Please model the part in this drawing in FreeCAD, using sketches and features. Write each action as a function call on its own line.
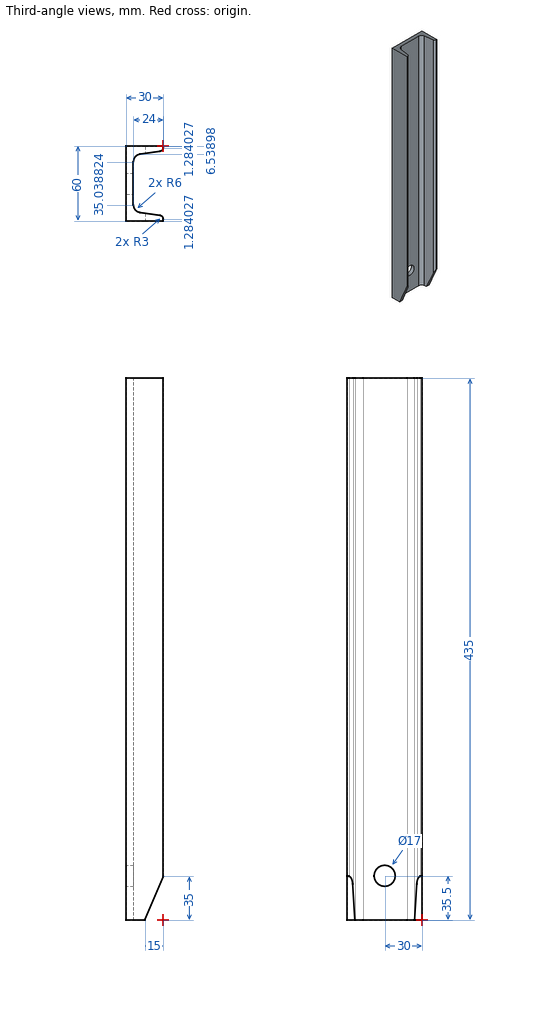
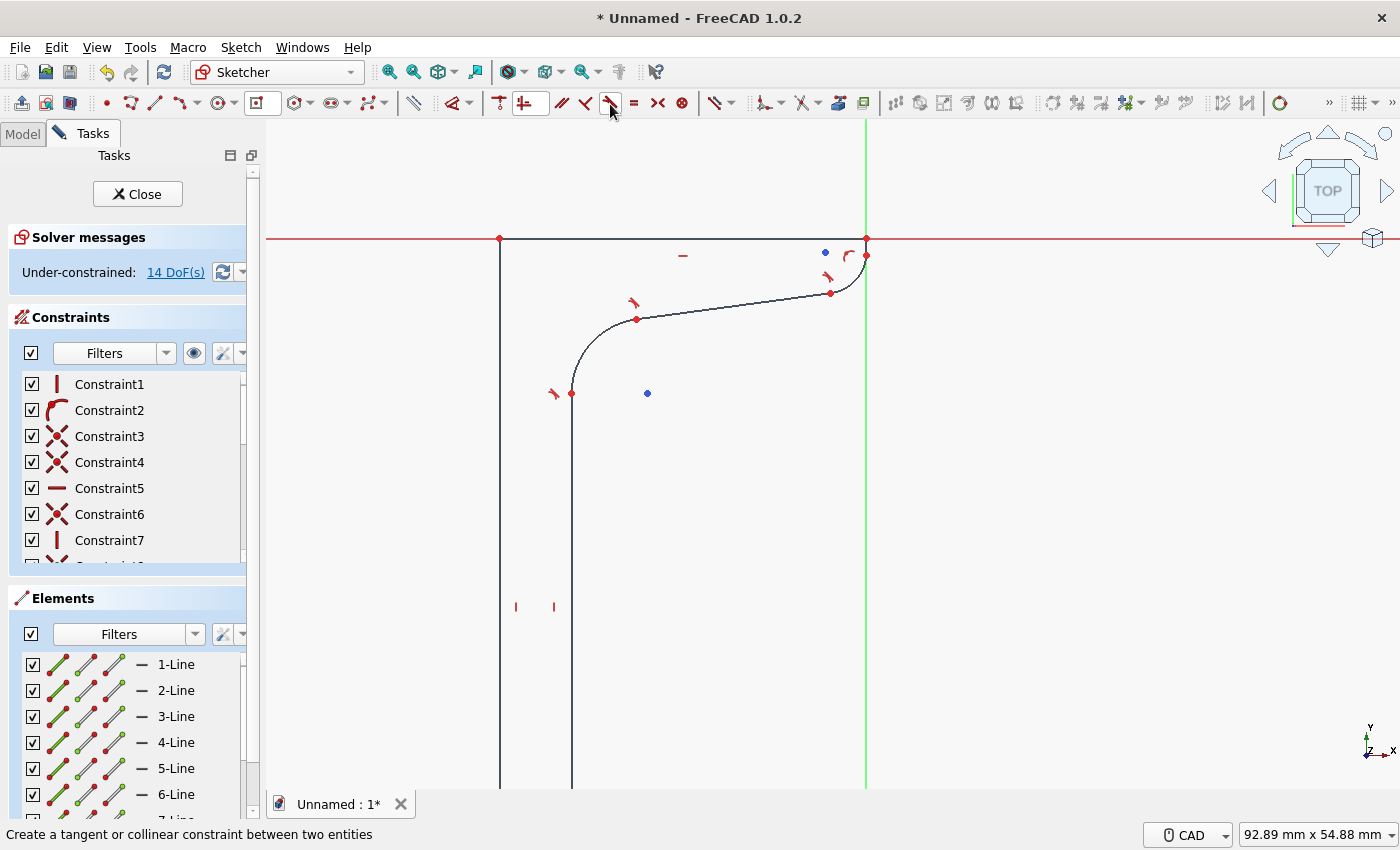
scroll(866, 247, up, 3)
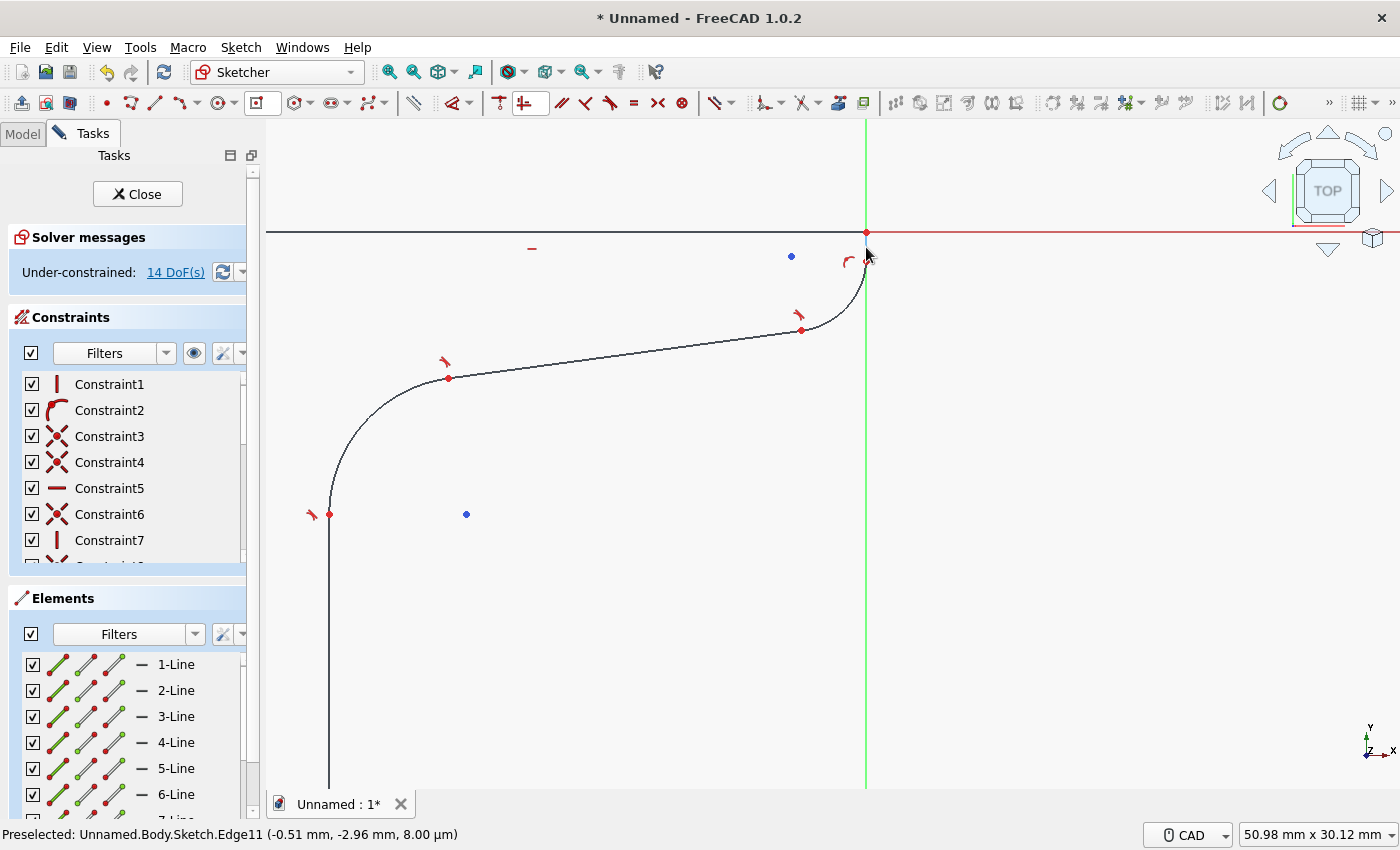
click(866, 247)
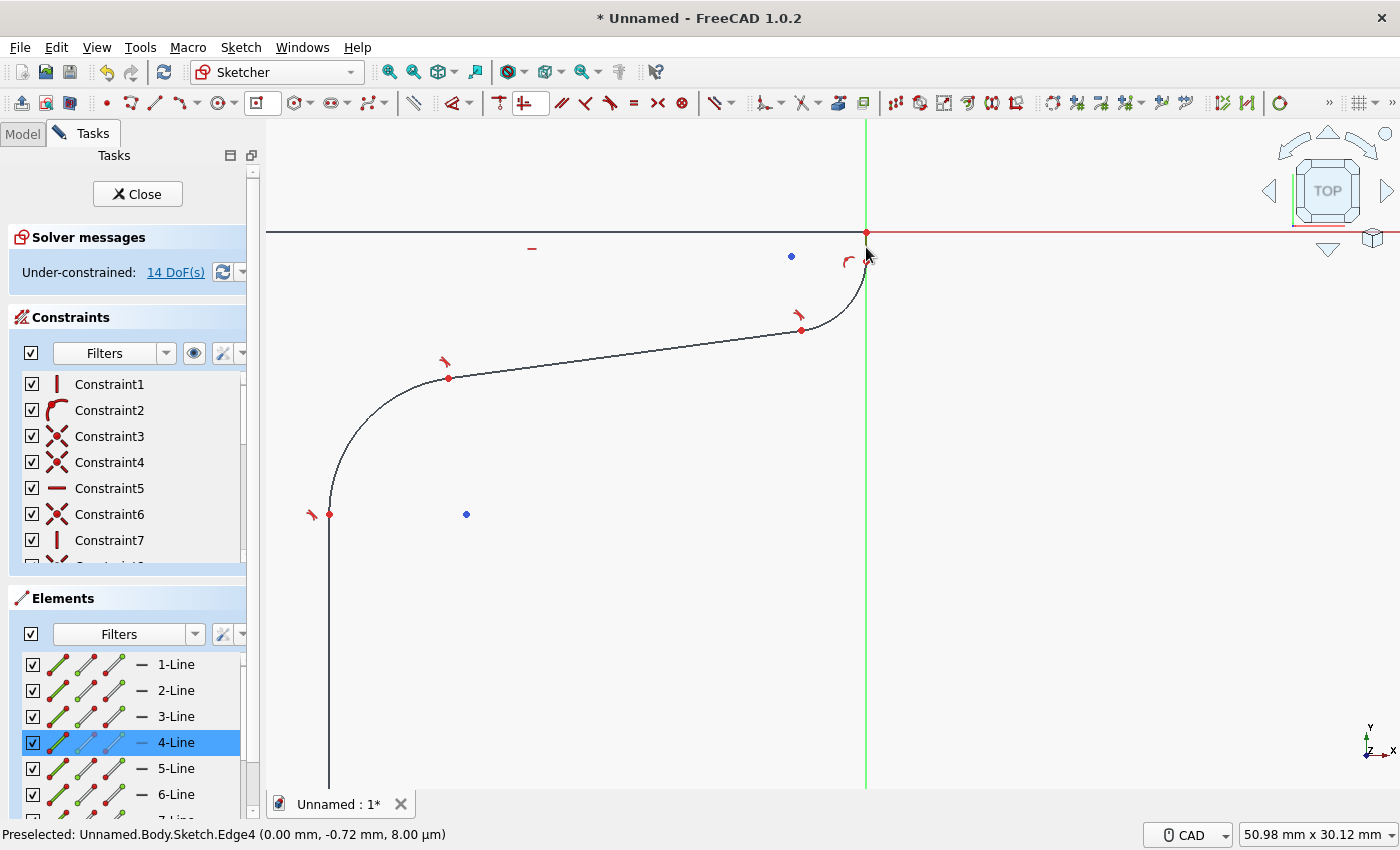
click(831, 321)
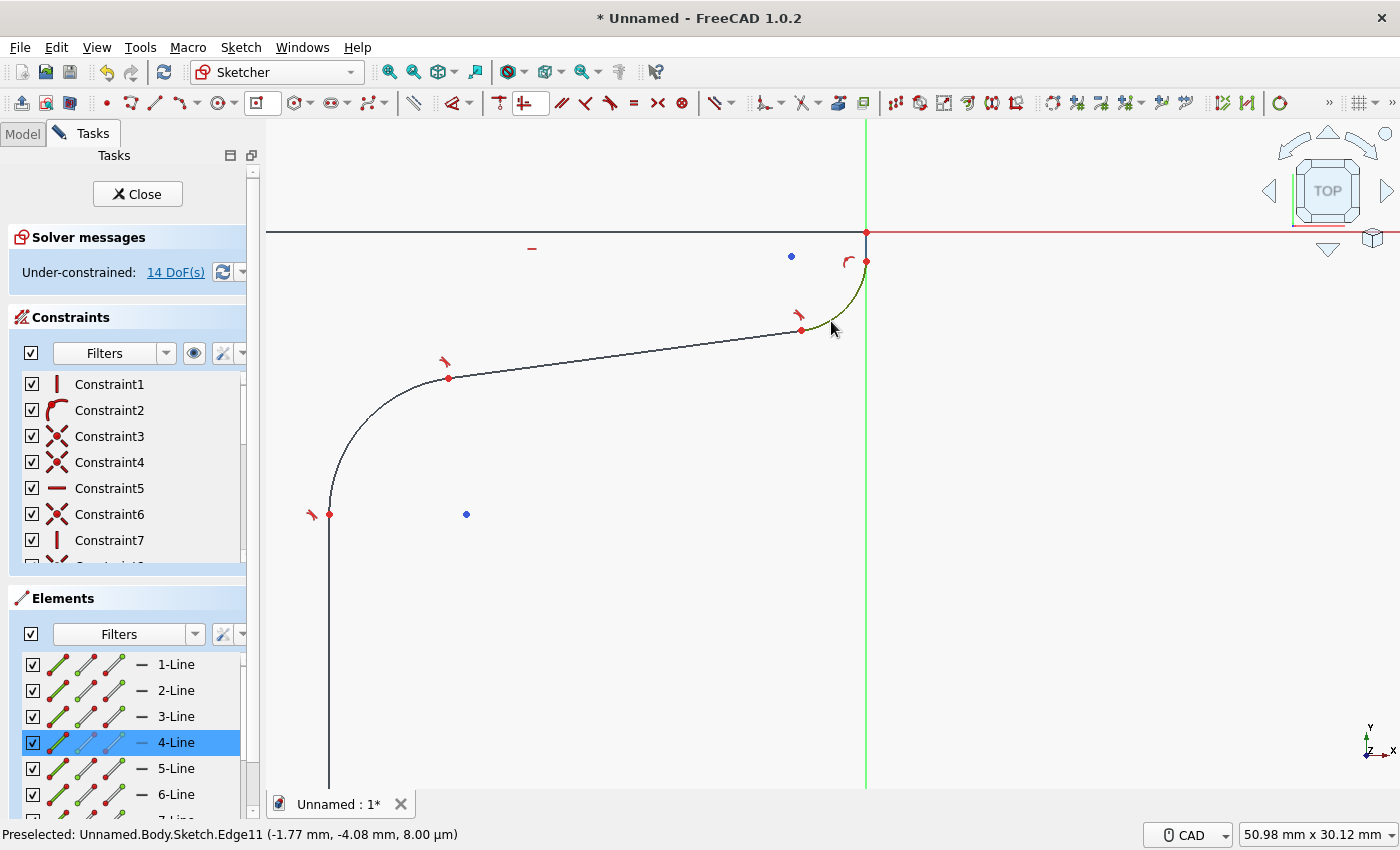
key(t)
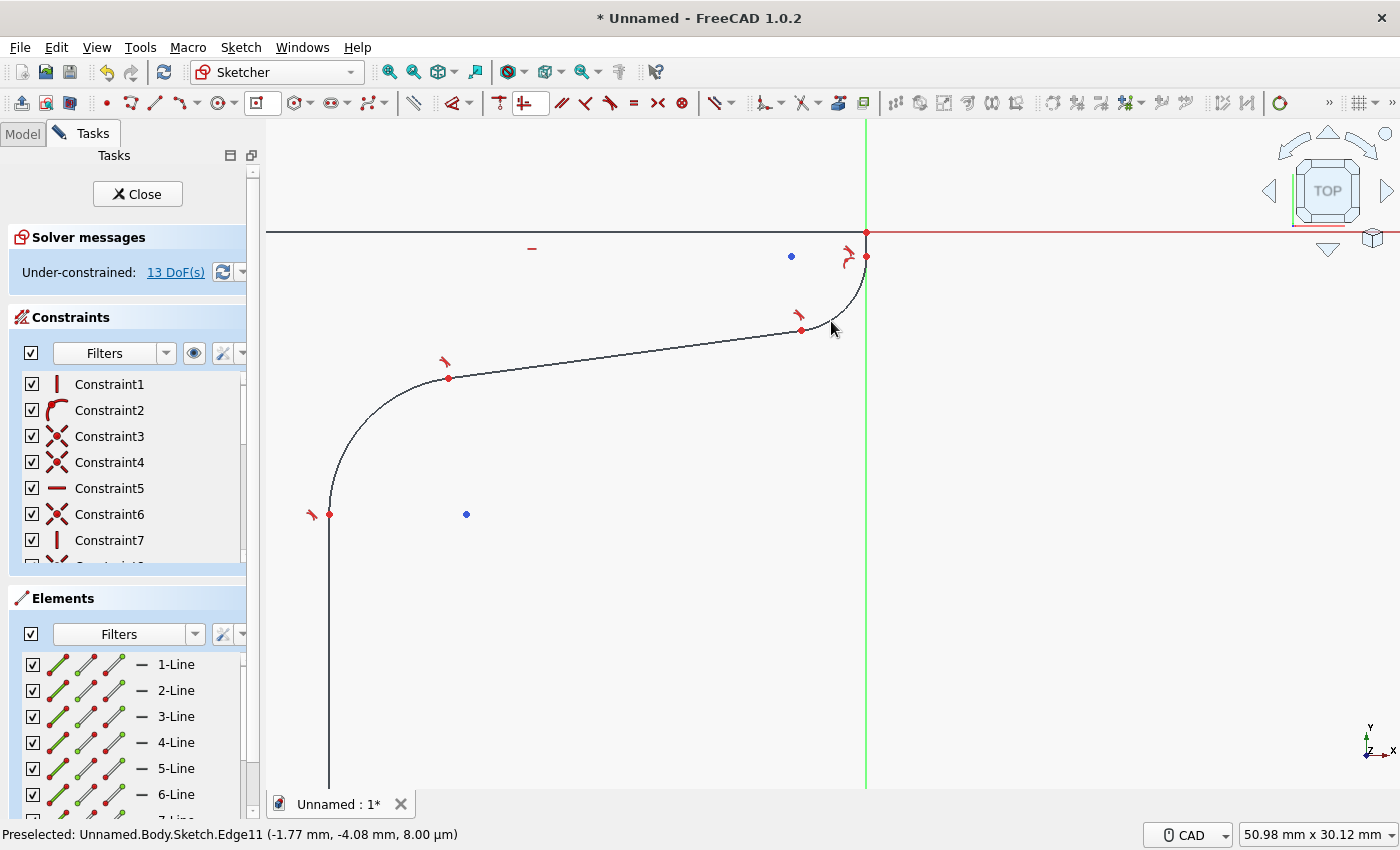
scroll(864, 262, down, 6)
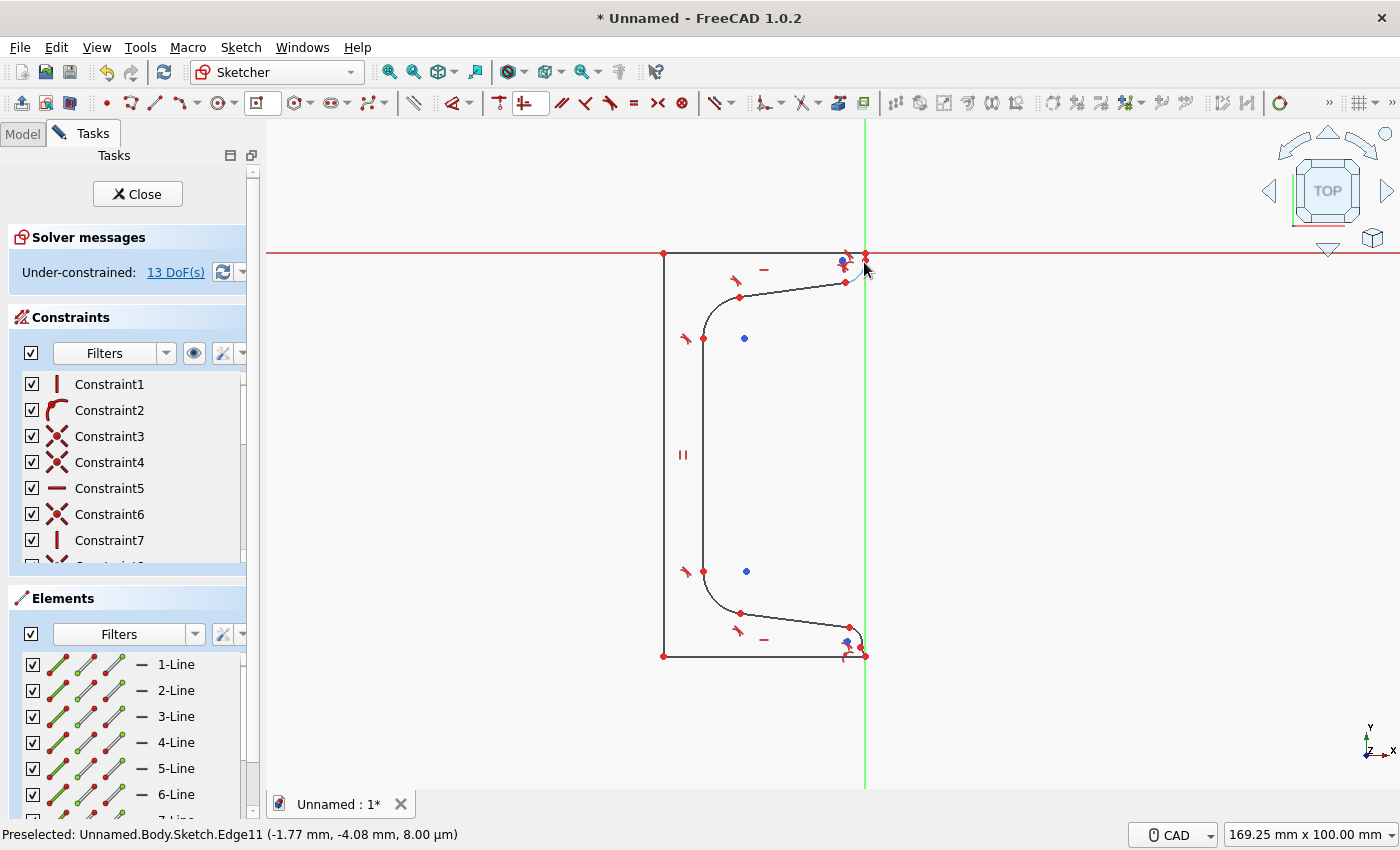
scroll(862, 650, up, 8)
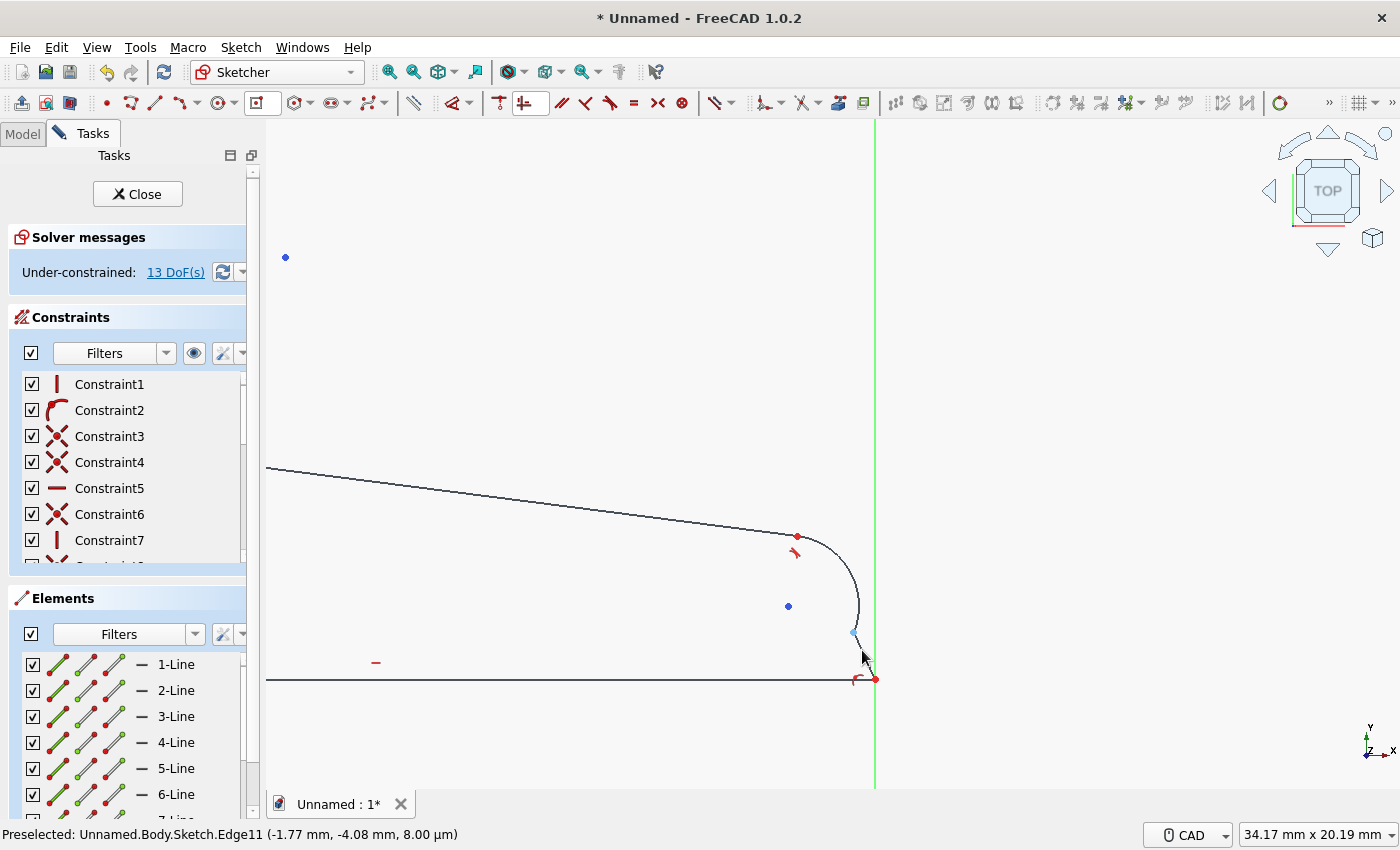
click(860, 647)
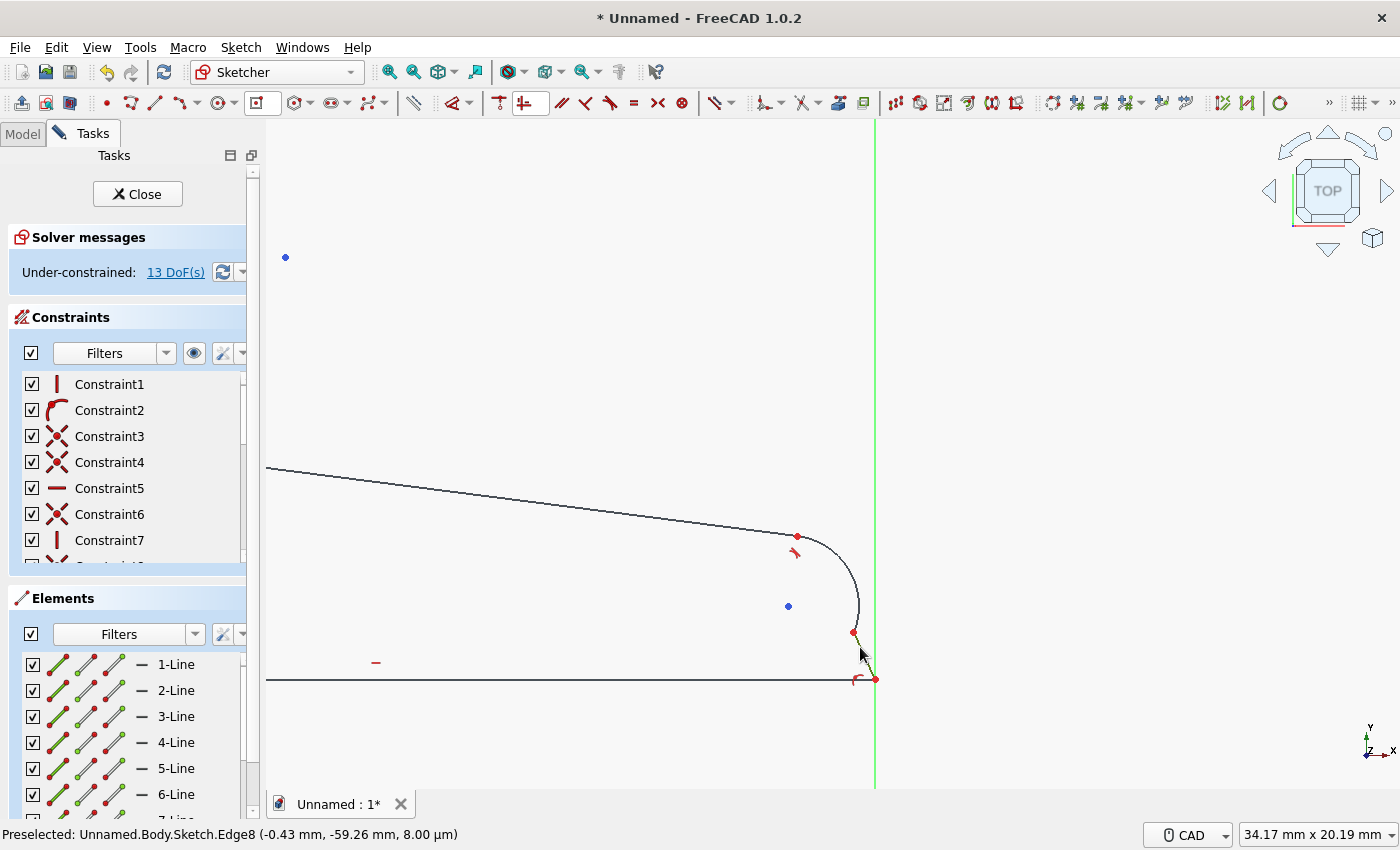
click(858, 594)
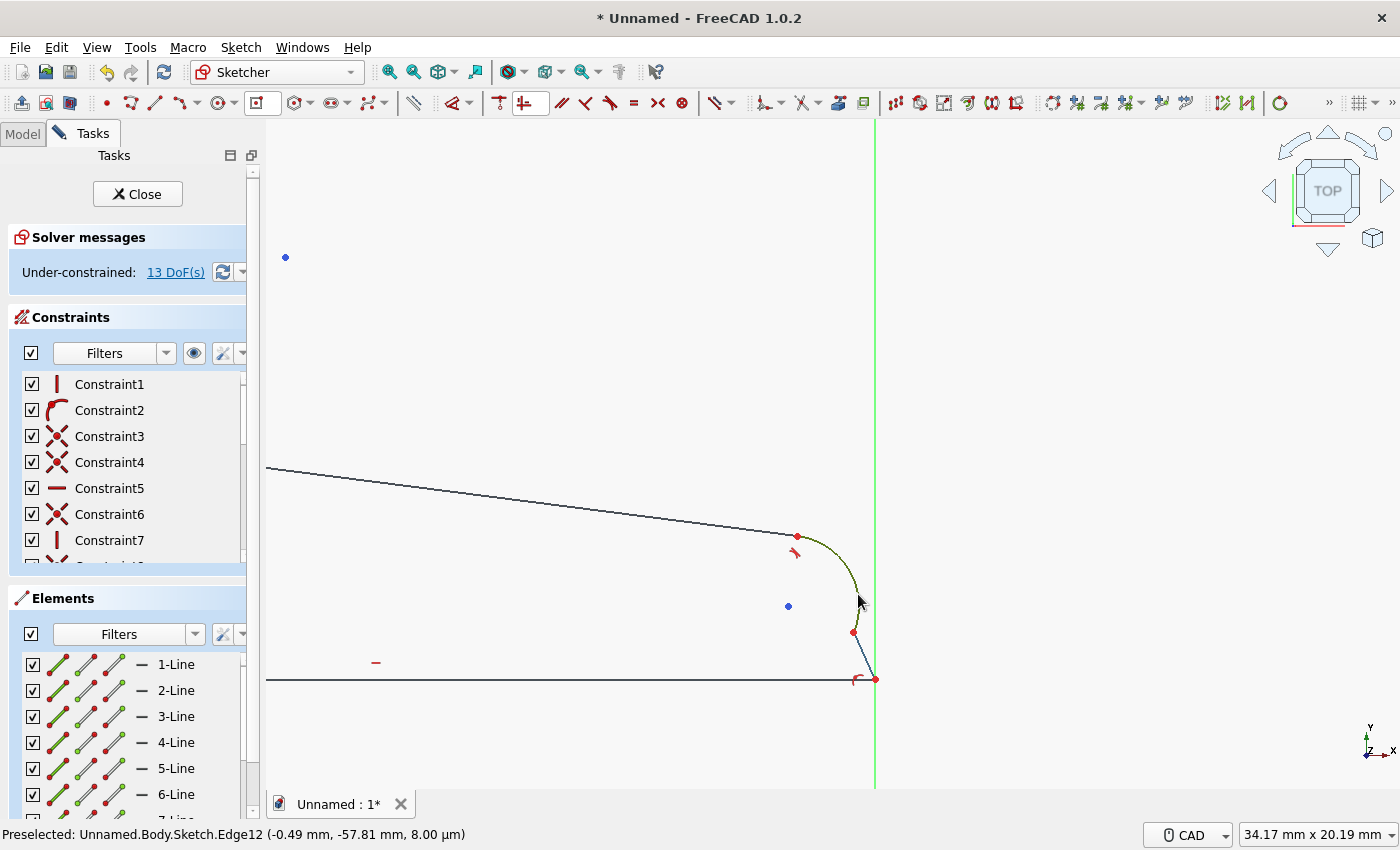
click(610, 104)